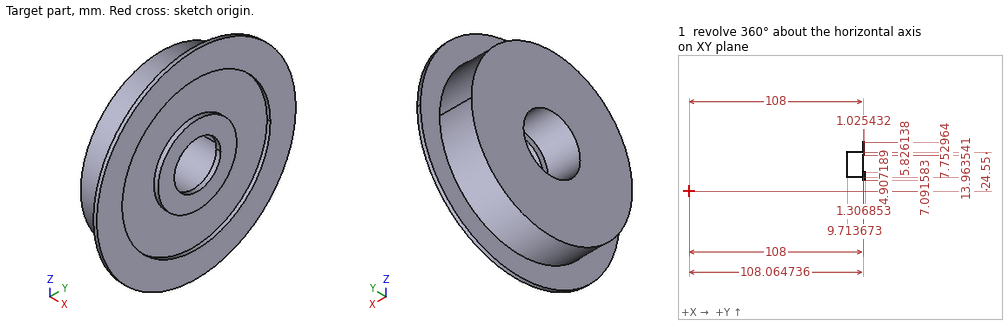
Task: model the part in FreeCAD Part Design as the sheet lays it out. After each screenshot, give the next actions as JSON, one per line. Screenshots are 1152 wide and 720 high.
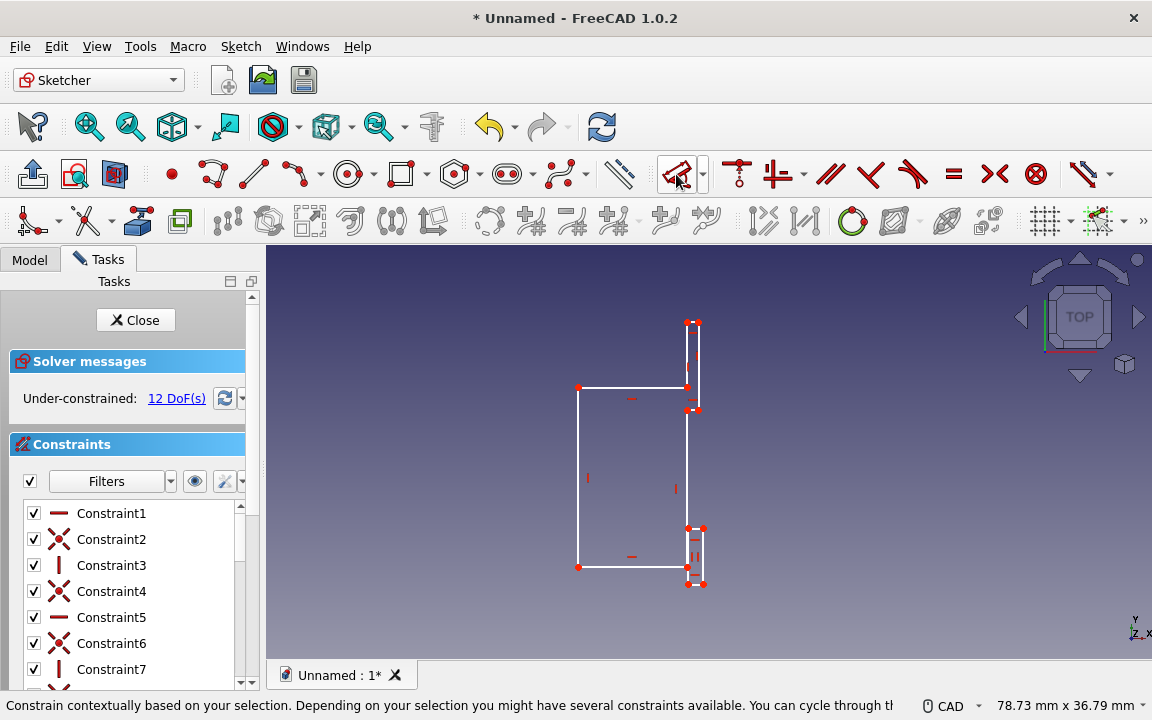
{"action": "left_click", "coordinate": [687, 567]}
{"action": "left_click", "coordinate": [491, 533]}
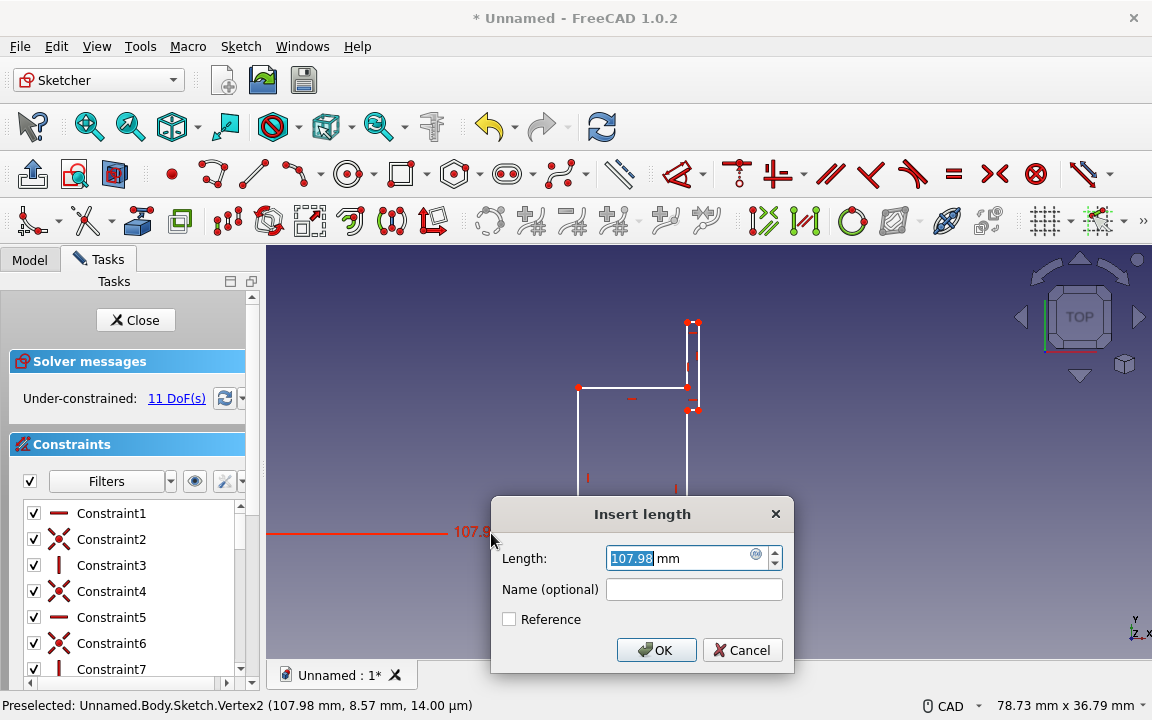
{"action": "type", "text": "108"}
{"action": "key", "text": "Return"}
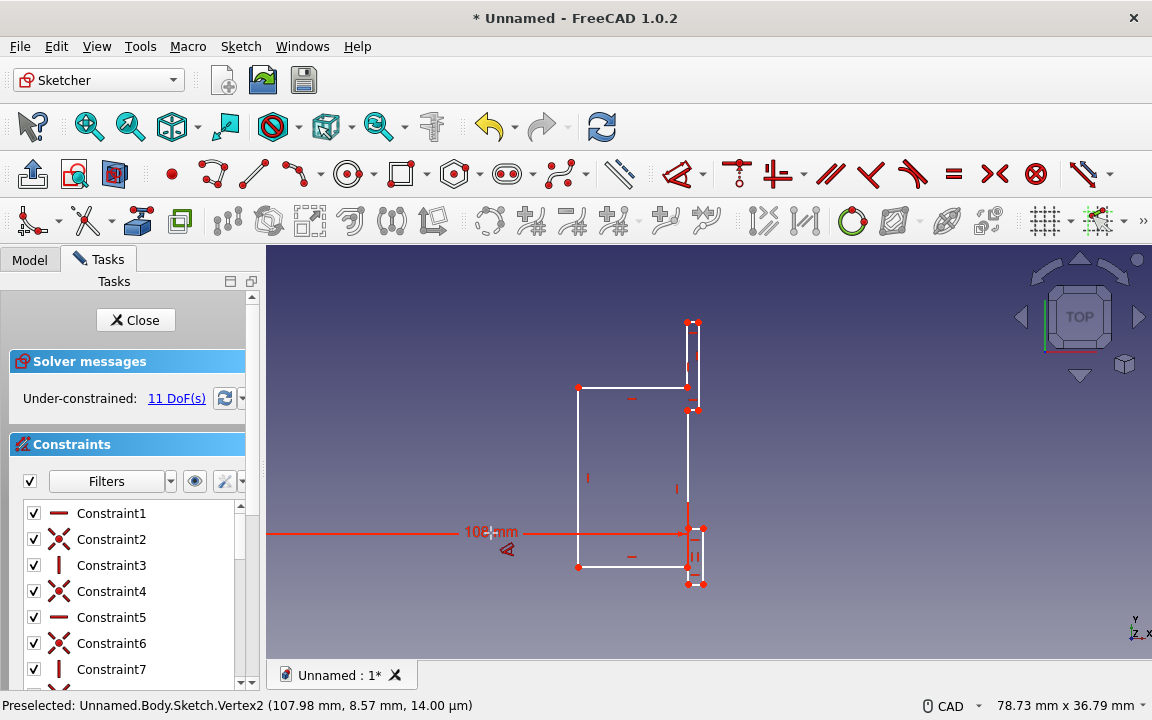
{"action": "left_click", "coordinate": [687, 322]}
{"action": "left_click", "coordinate": [491, 288]}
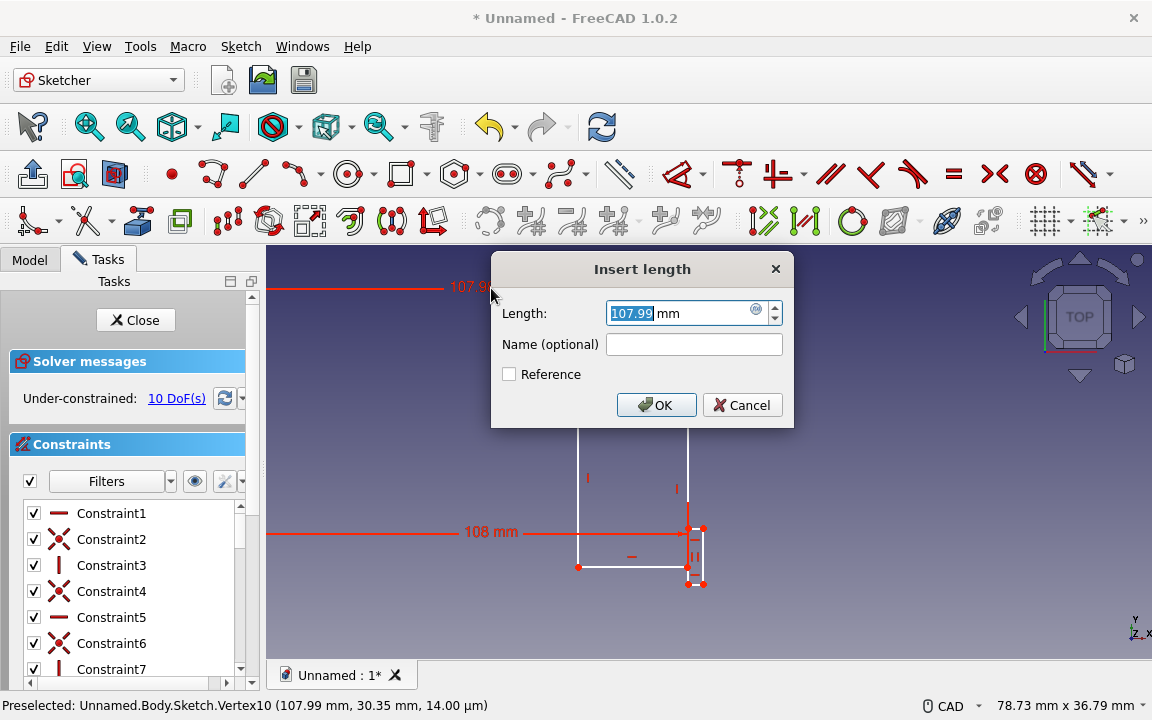
{"action": "type", "text": "108"}
{"action": "key", "text": "Return"}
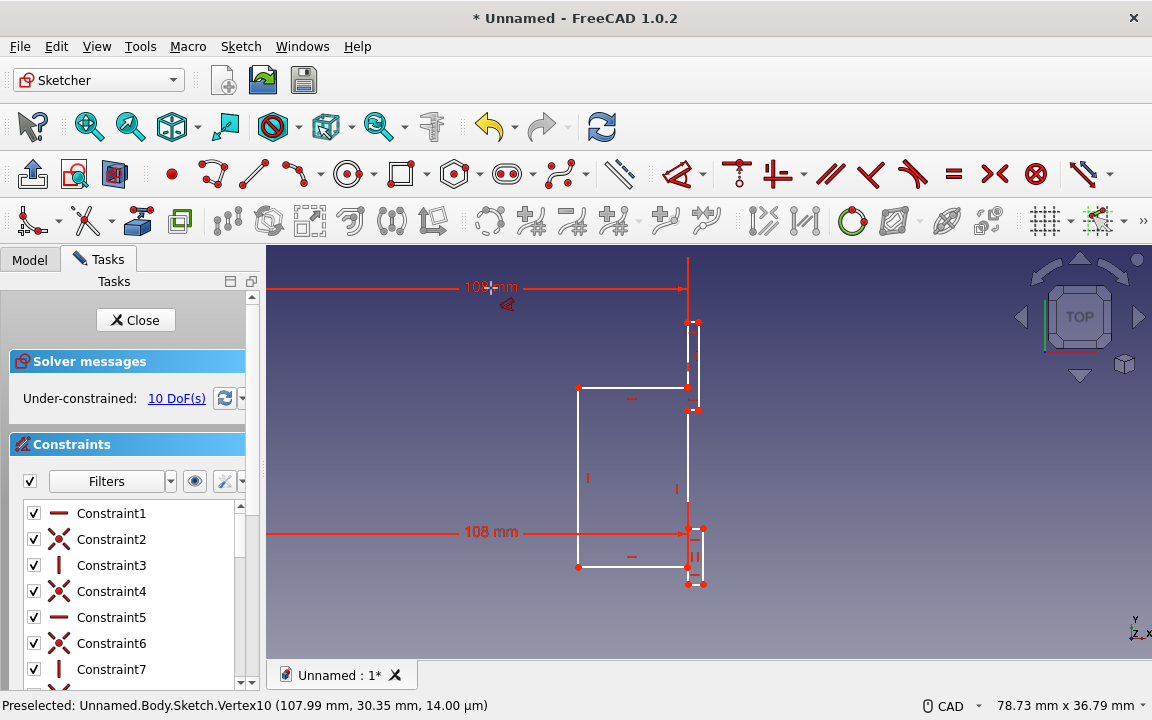
{"action": "left_click", "coordinate": [688, 388]}
{"action": "left_click", "coordinate": [722, 509]}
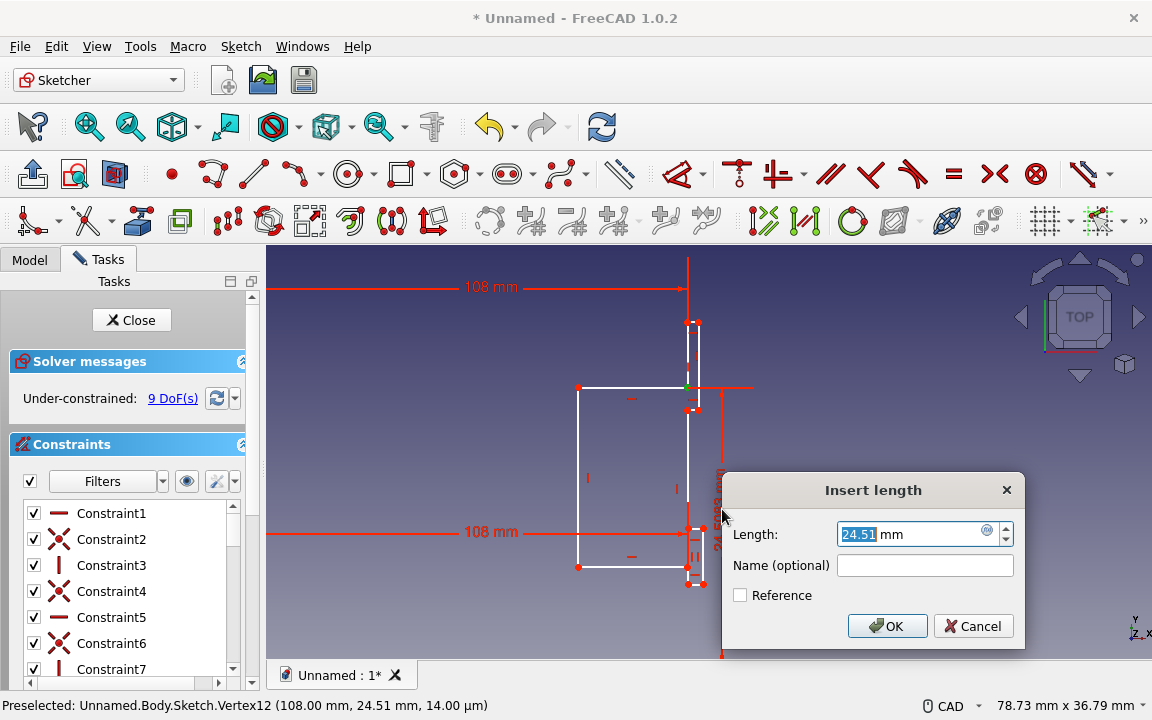
{"action": "type", "text": "24.55"}
{"action": "key", "text": "Return"}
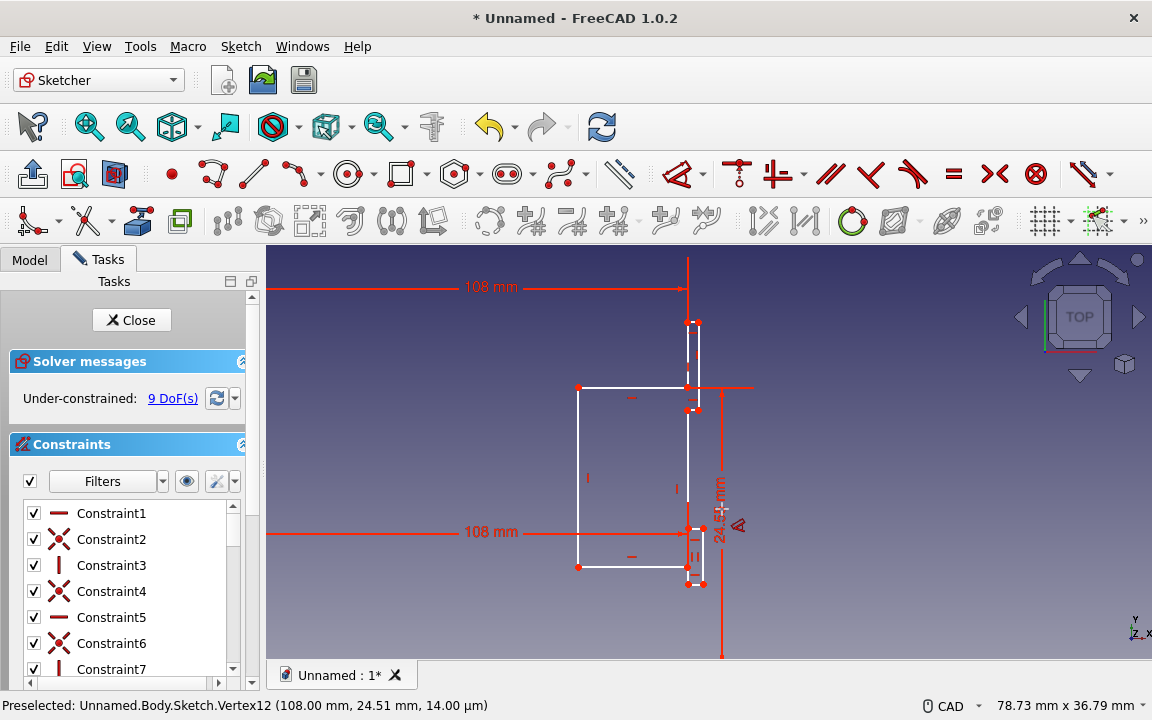
{"action": "left_click", "coordinate": [611, 567]}
{"action": "left_click", "coordinate": [633, 601]}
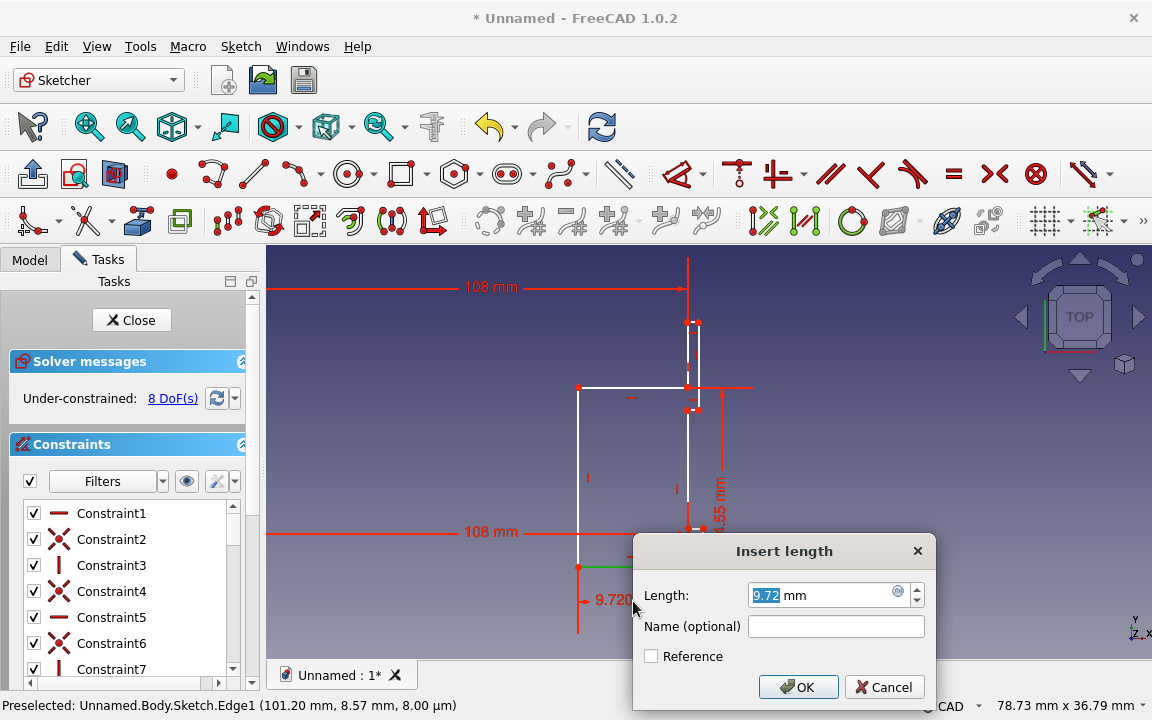
{"action": "type", "text": "9.713673"}
{"action": "key", "text": "Return"}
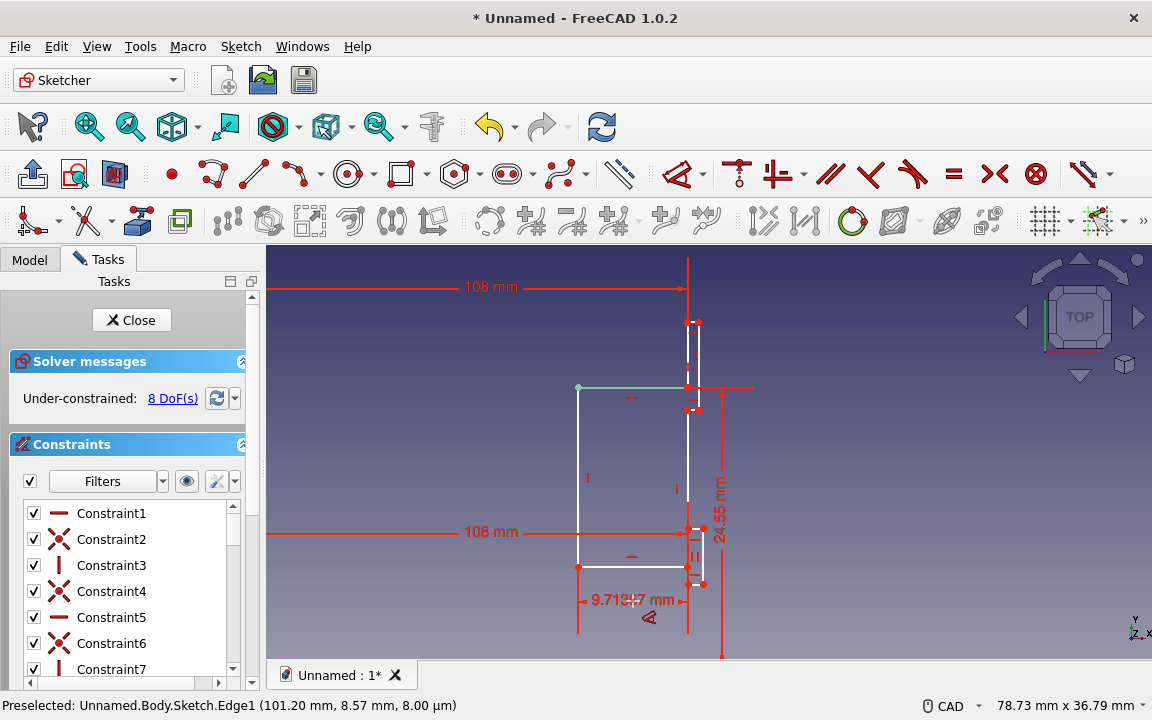
{"action": "scroll", "coordinate": [693, 410], "scroll_direction": "up", "scroll_amount": 7}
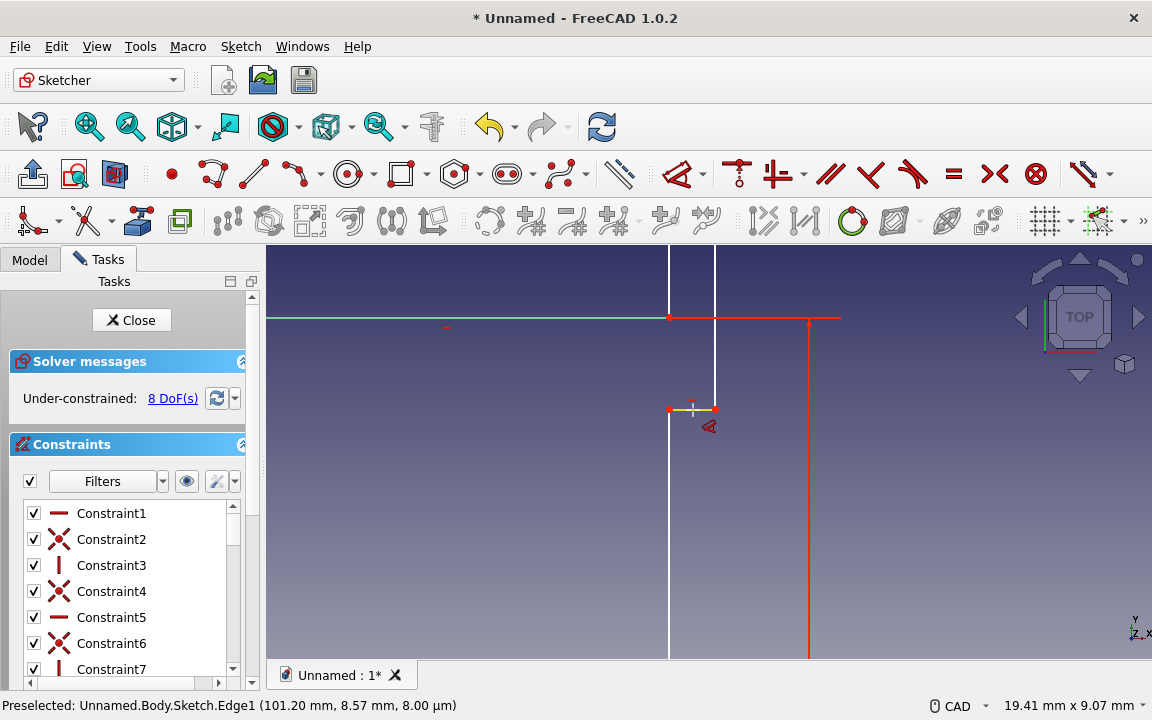
{"action": "left_click", "coordinate": [692, 410]}
{"action": "left_click", "coordinate": [692, 376]}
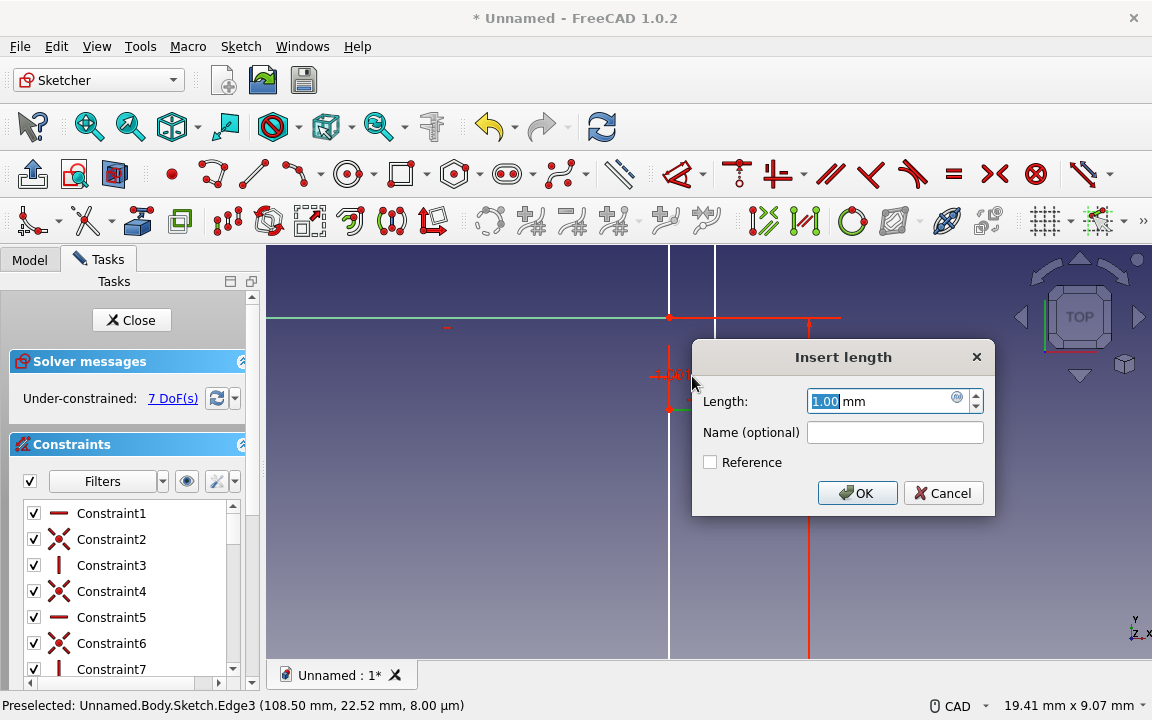
{"action": "type", "text": "1.025432"}
{"action": "key", "text": "Return"}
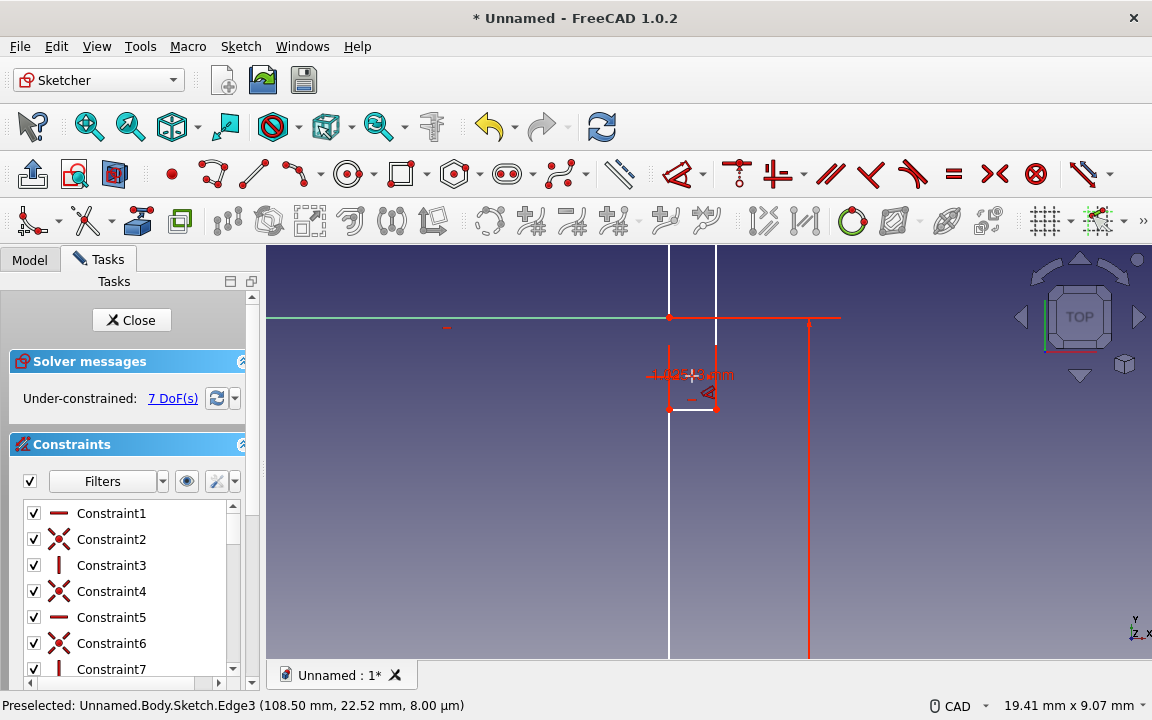
{"action": "scroll", "coordinate": [693, 409], "scroll_direction": "down", "scroll_amount": 7}